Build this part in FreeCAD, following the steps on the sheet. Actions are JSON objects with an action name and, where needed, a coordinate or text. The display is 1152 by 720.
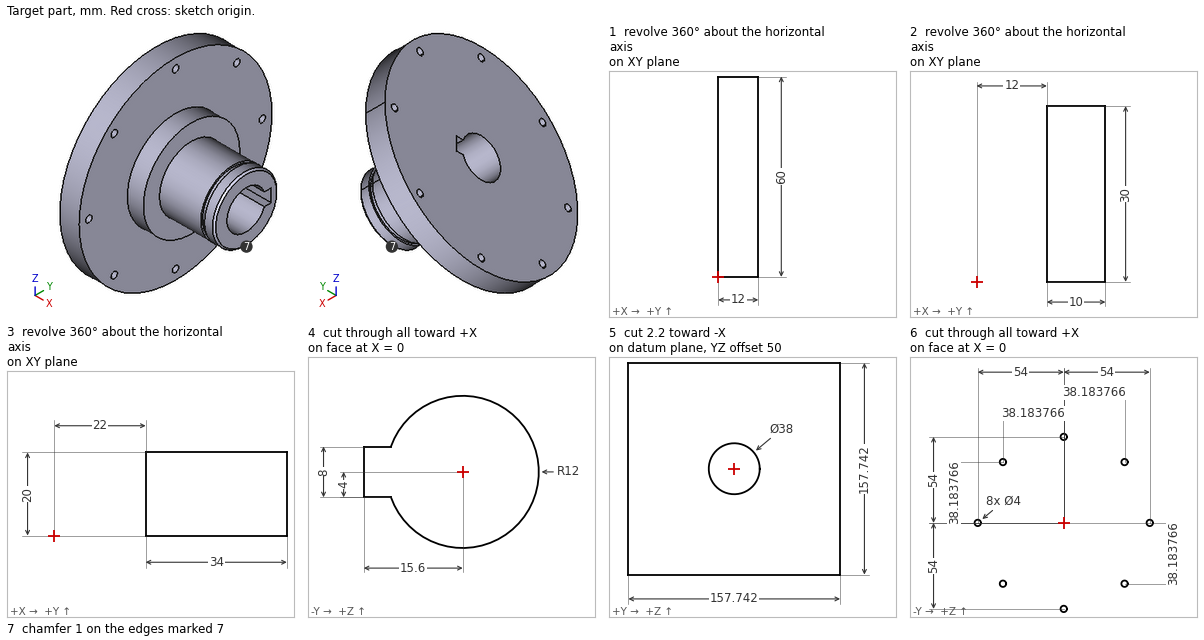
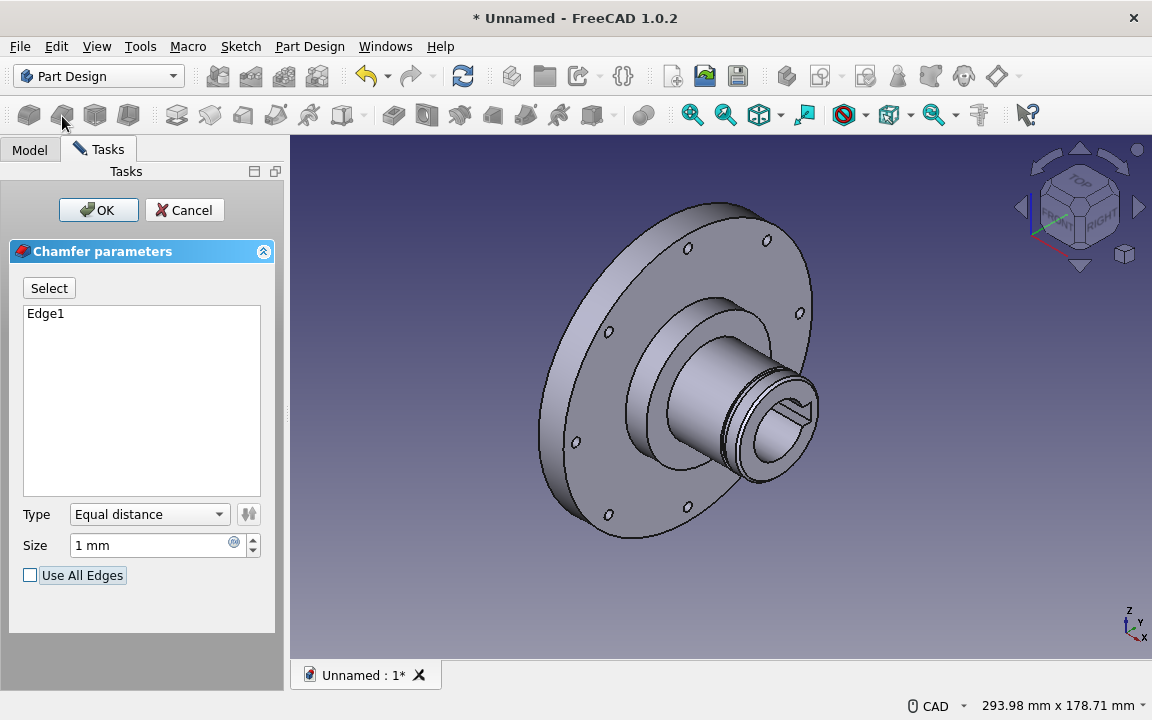
{"action": "left_click", "coordinate": [99, 210]}